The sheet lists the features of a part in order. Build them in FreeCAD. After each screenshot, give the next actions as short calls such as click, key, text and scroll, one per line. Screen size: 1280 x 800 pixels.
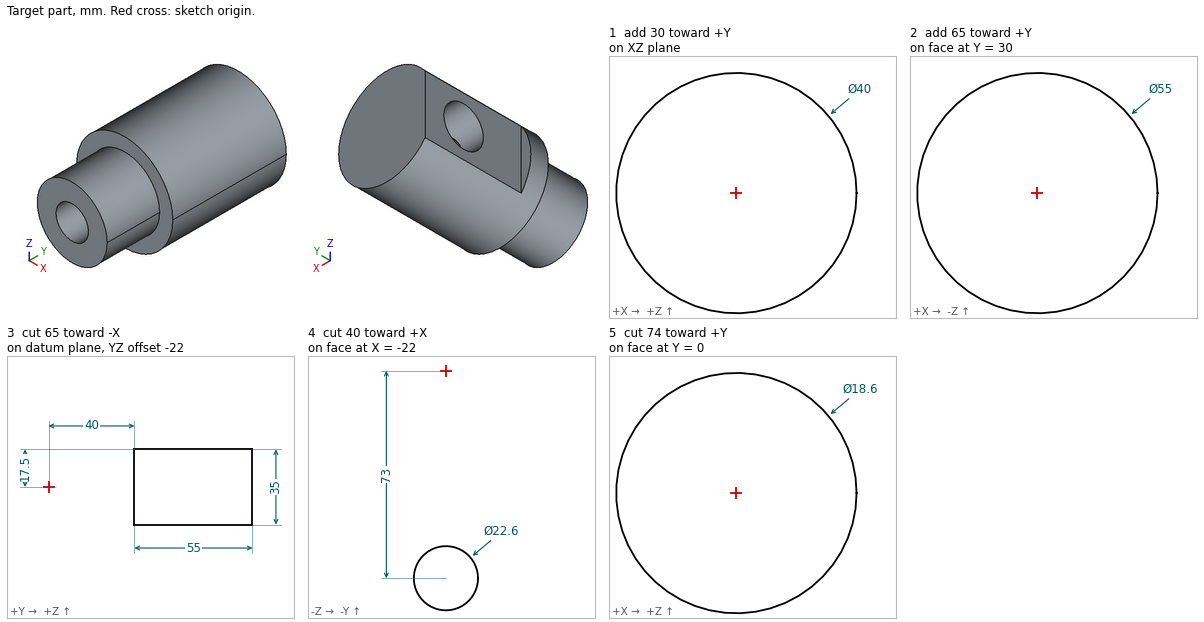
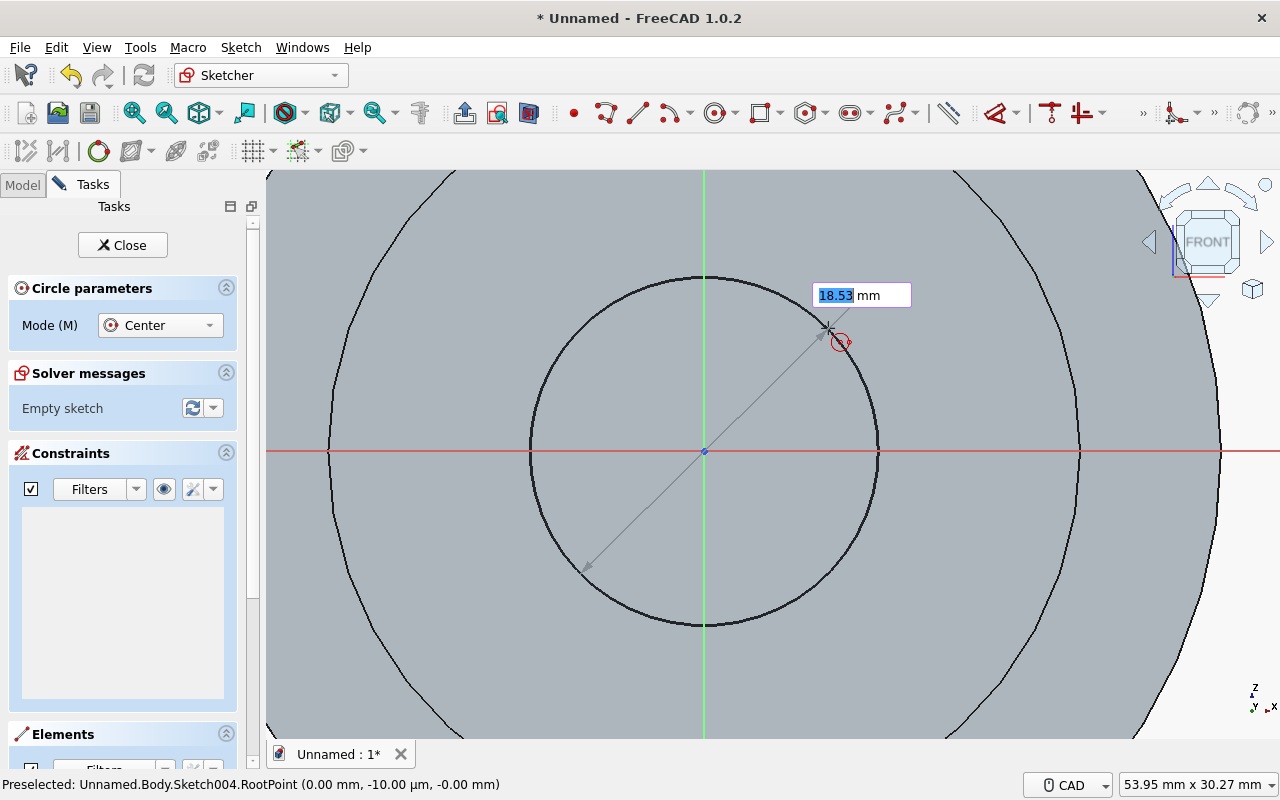
text(18.6)
key(Return)
key(Escape)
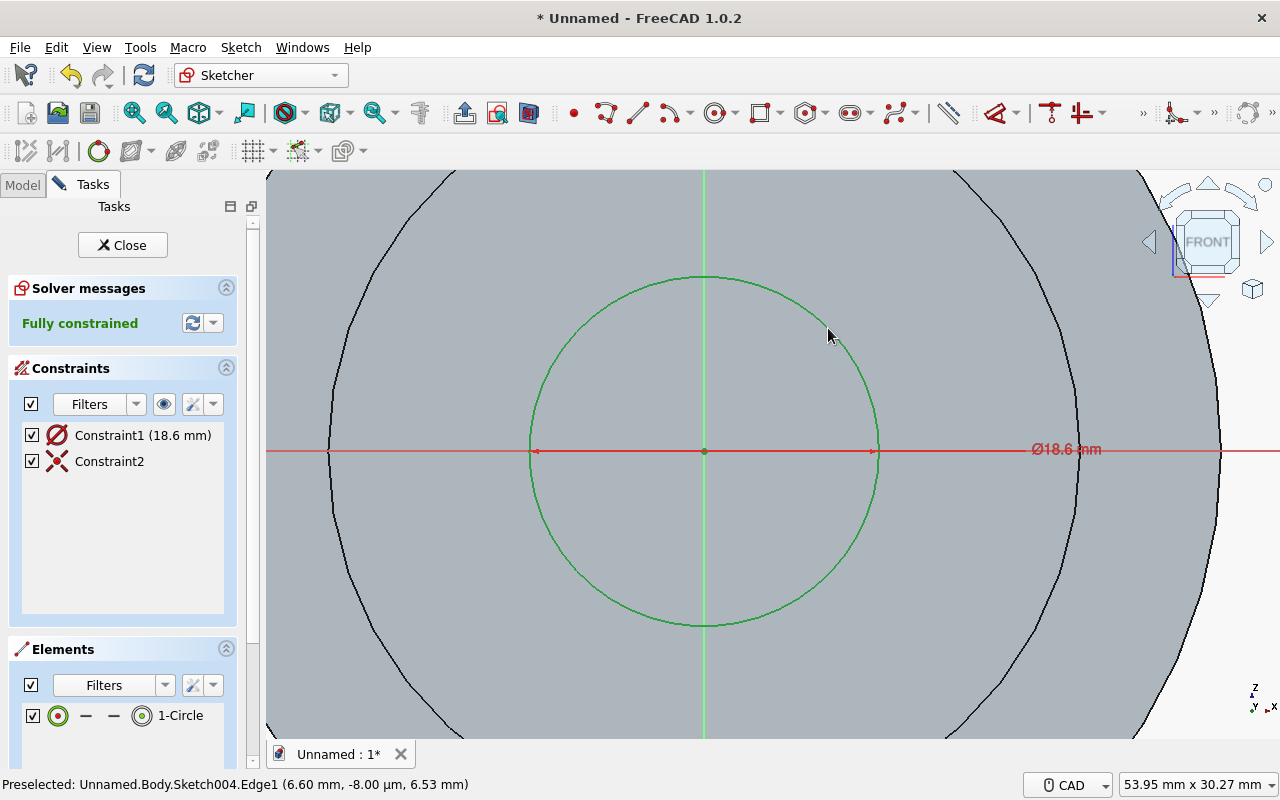
click(123, 245)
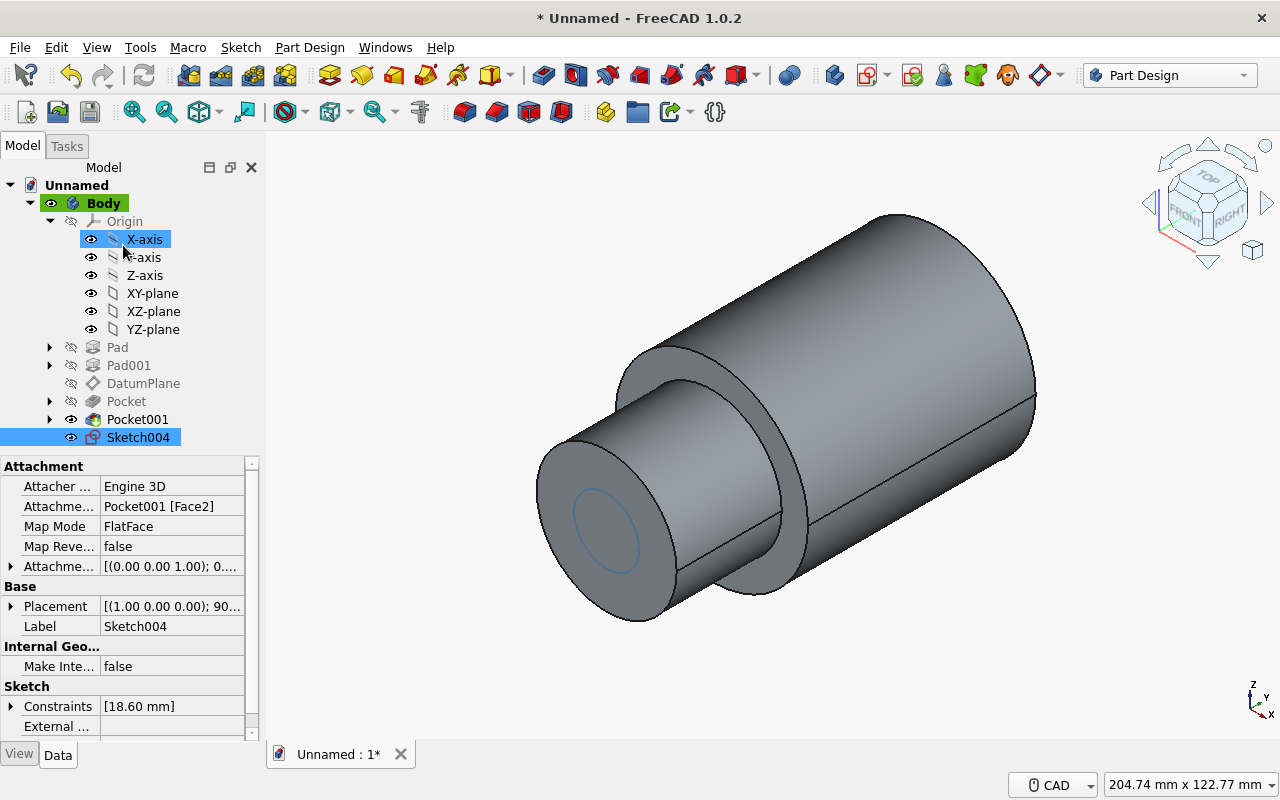
click(544, 76)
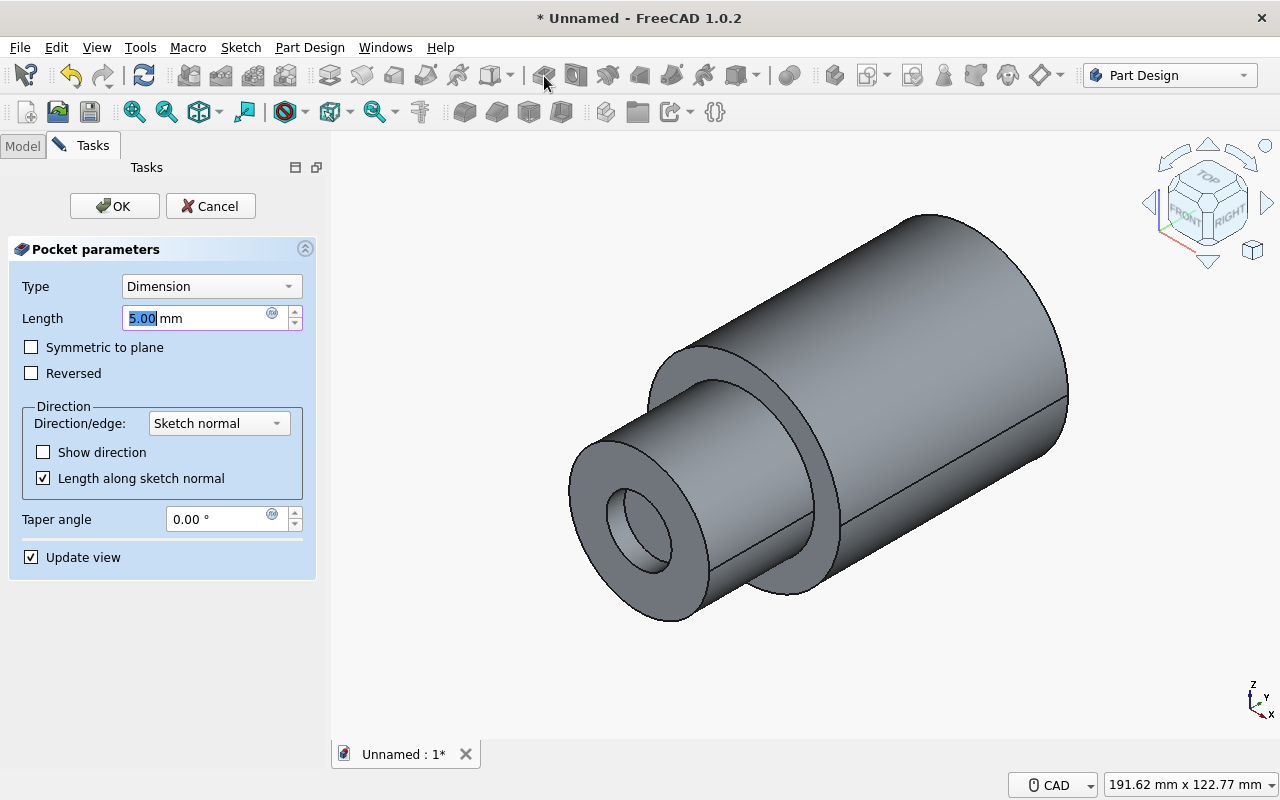
text(74)
key(Tab)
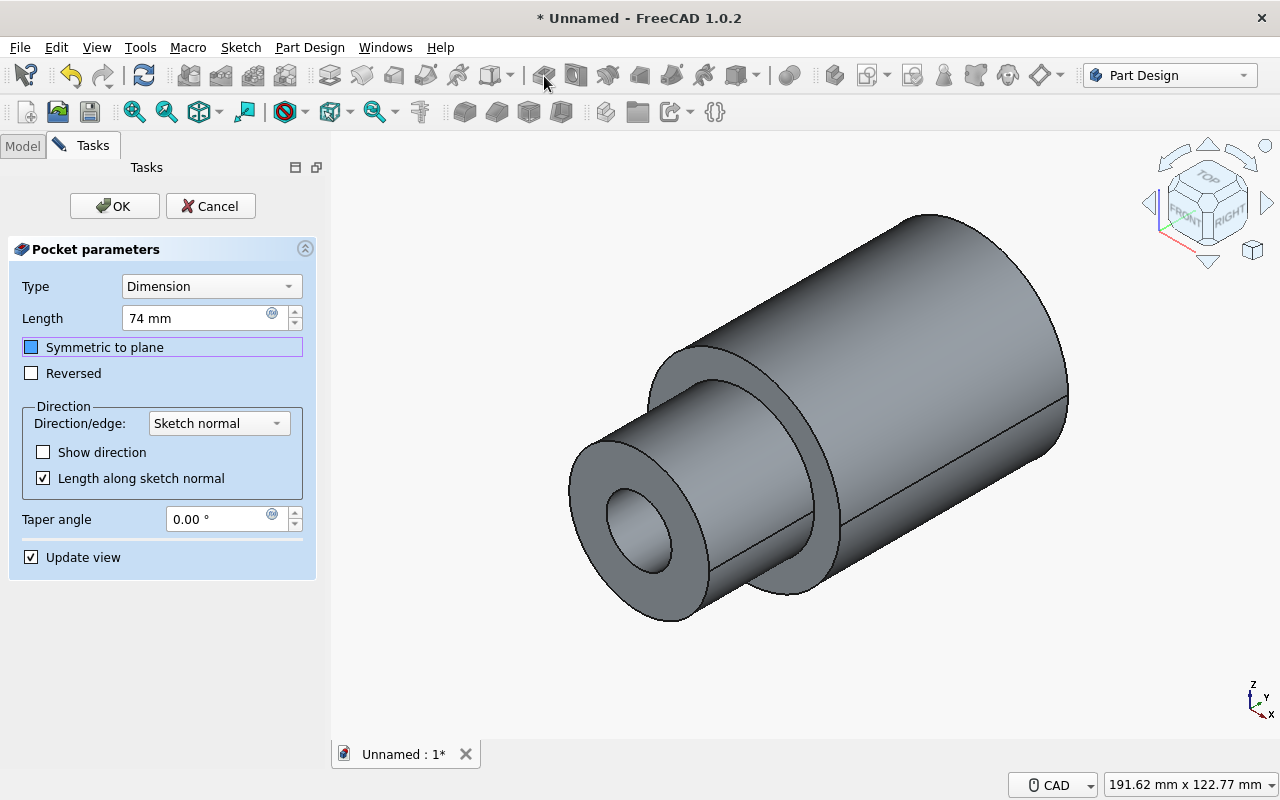
click(115, 206)